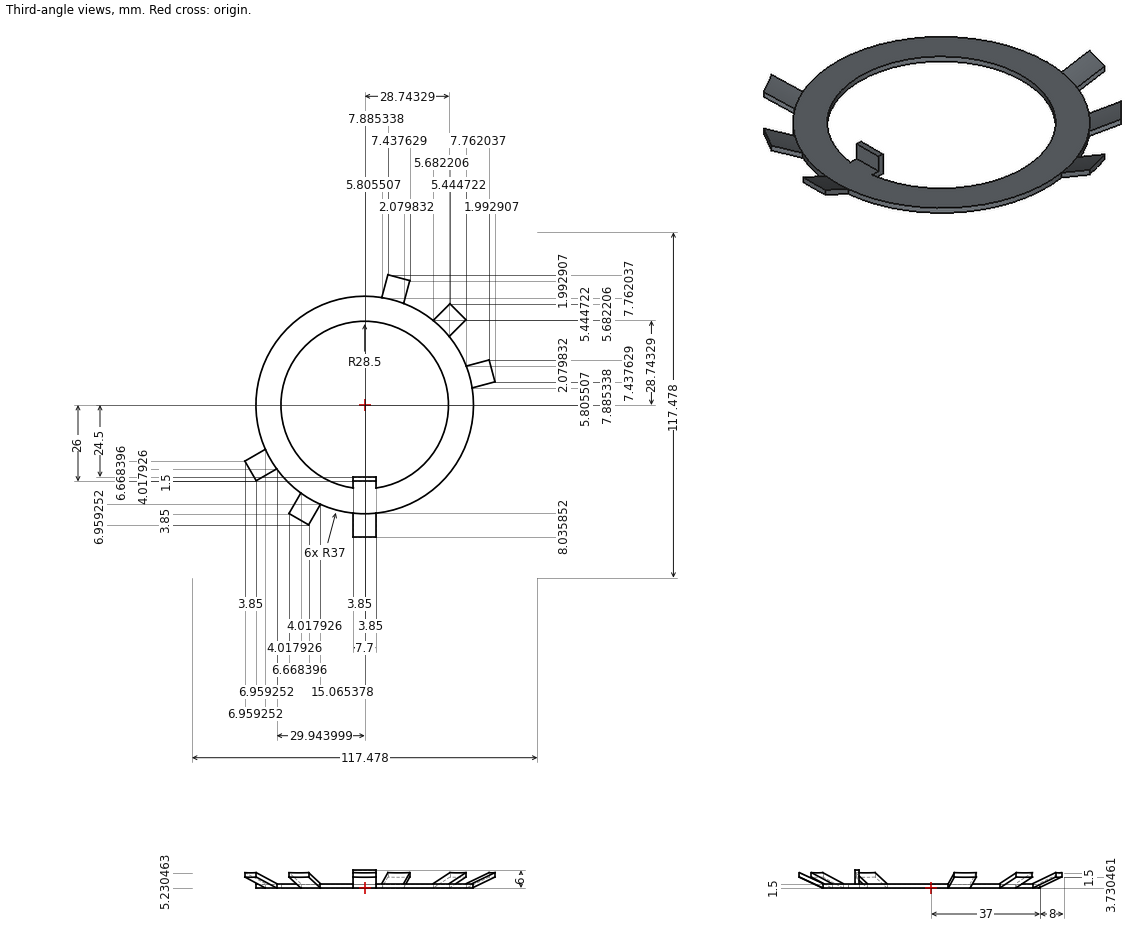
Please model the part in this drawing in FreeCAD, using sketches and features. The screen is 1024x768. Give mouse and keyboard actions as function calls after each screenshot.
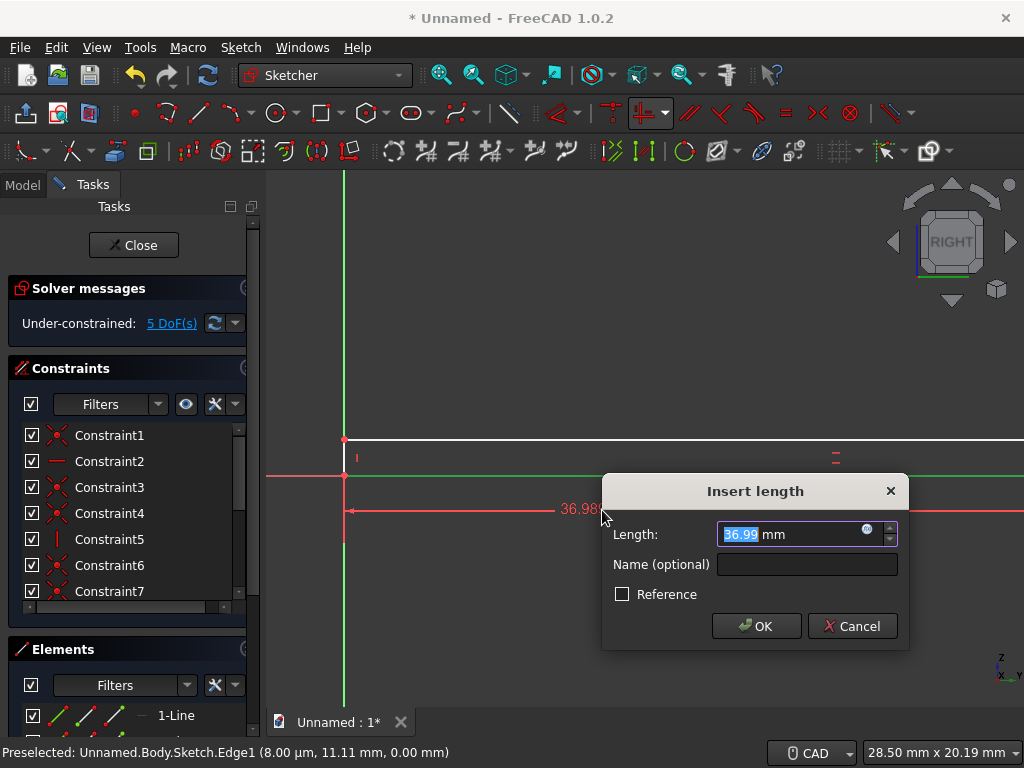
text(37)
key(Return)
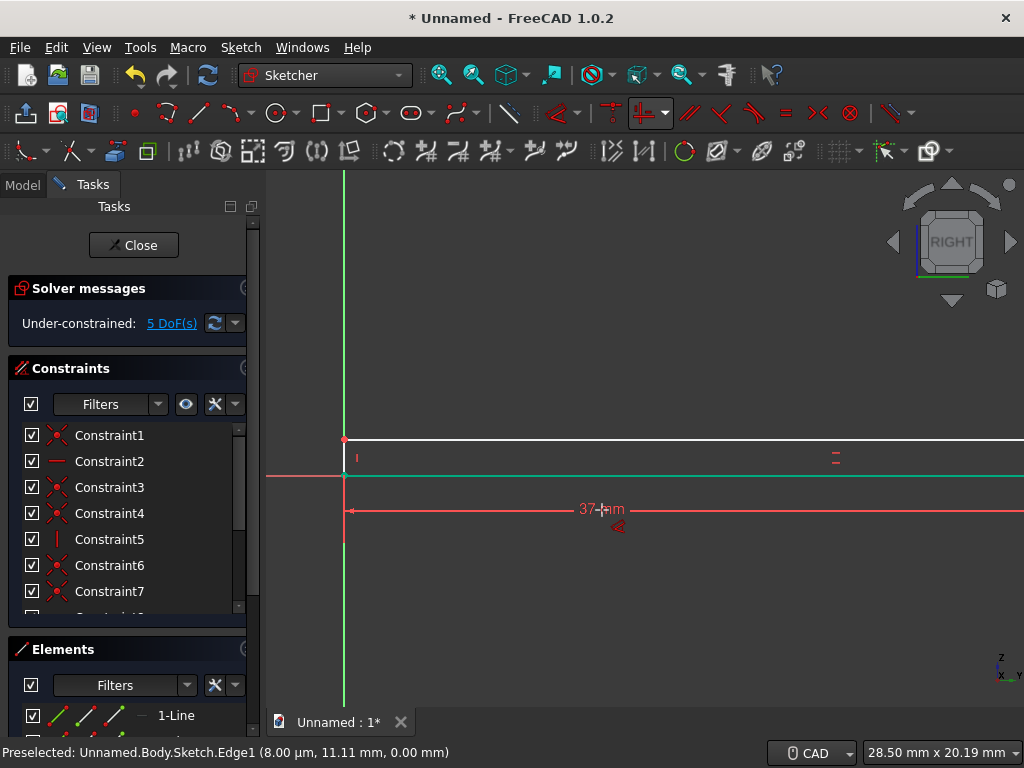
click(640, 439)
click(602, 405)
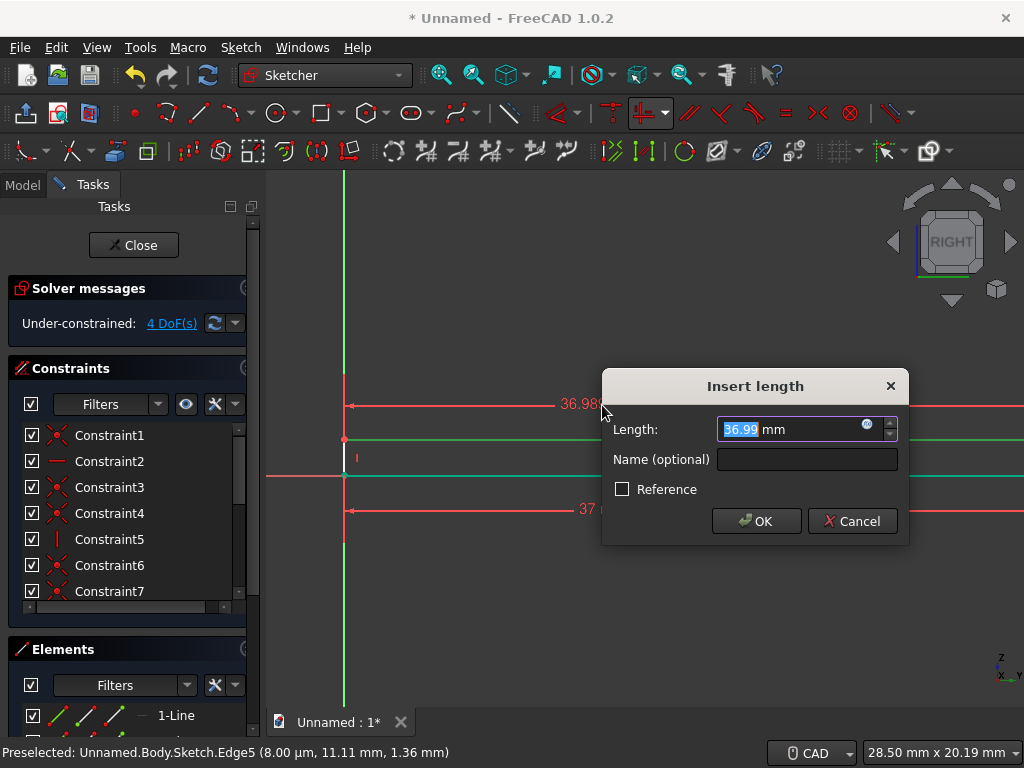
text(37)
key(Return)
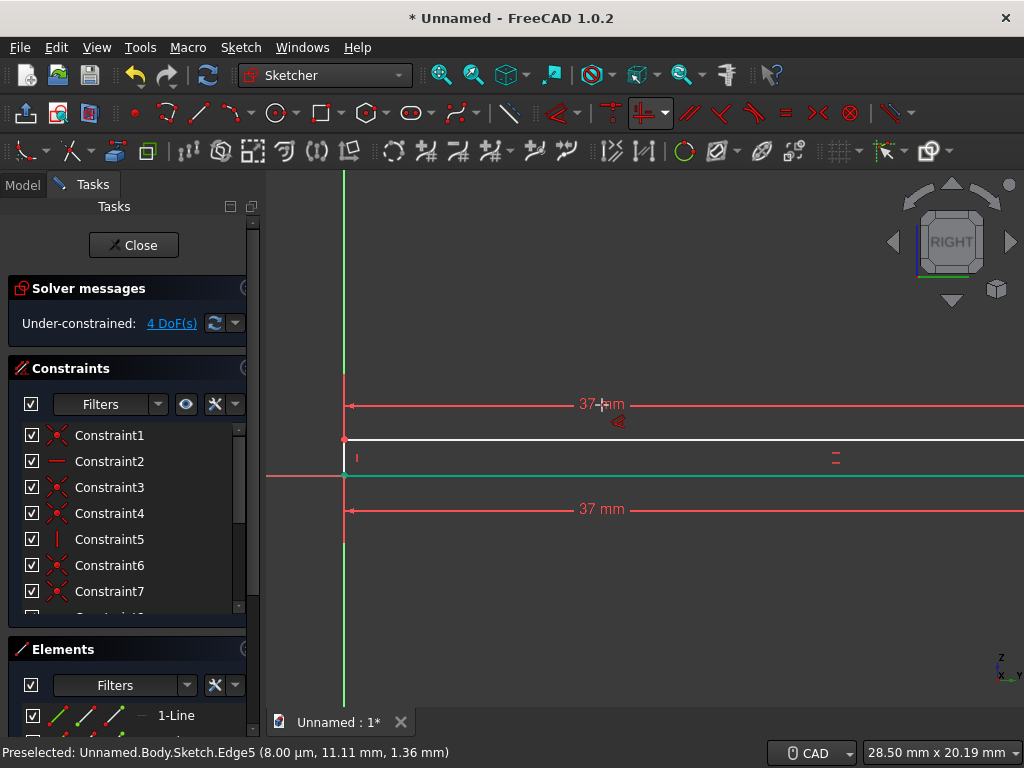
scroll(363, 457, down, 5)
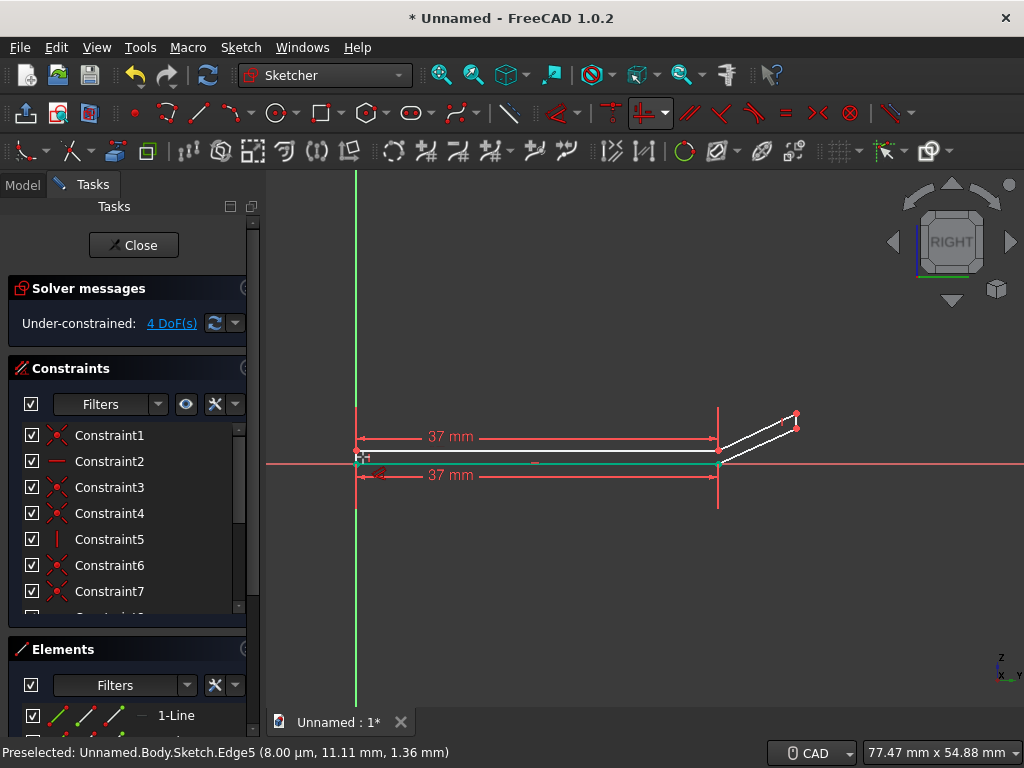
scroll(742, 454, up, 2)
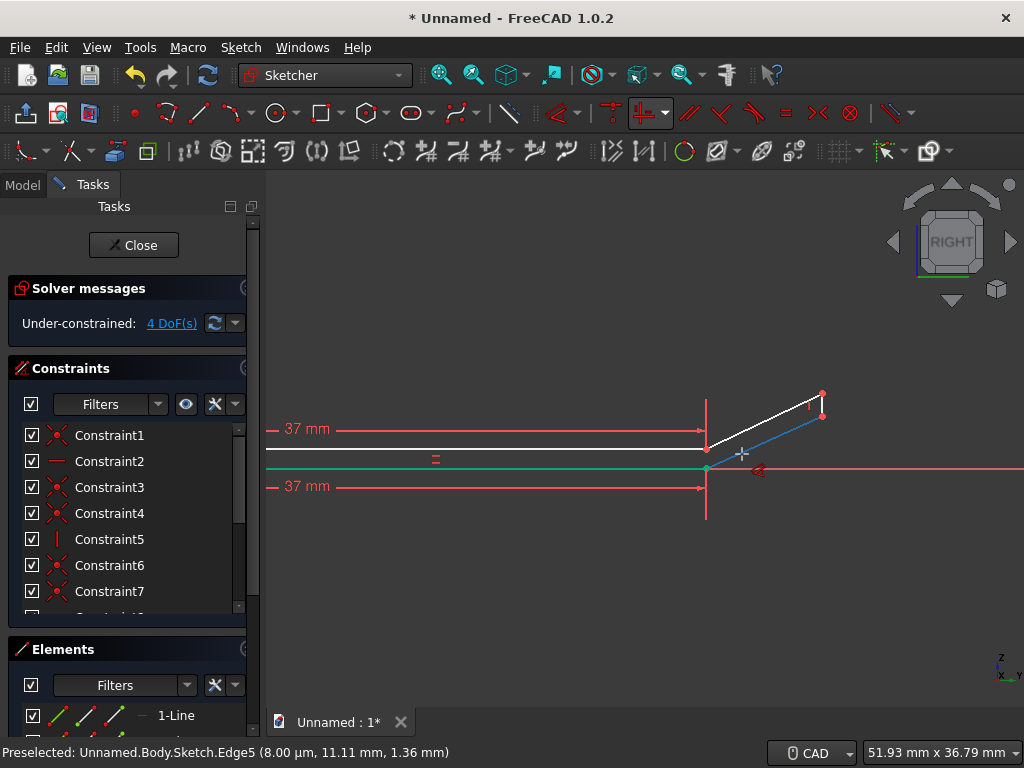
click(741, 453)
click(764, 503)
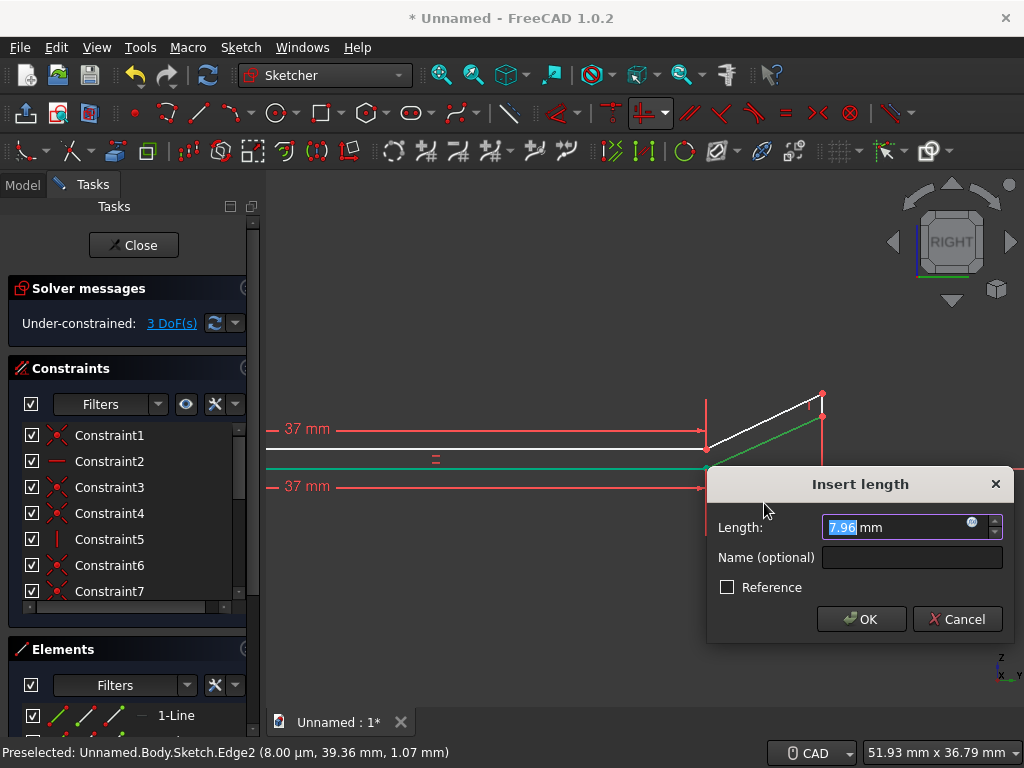
text(8)
key(Return)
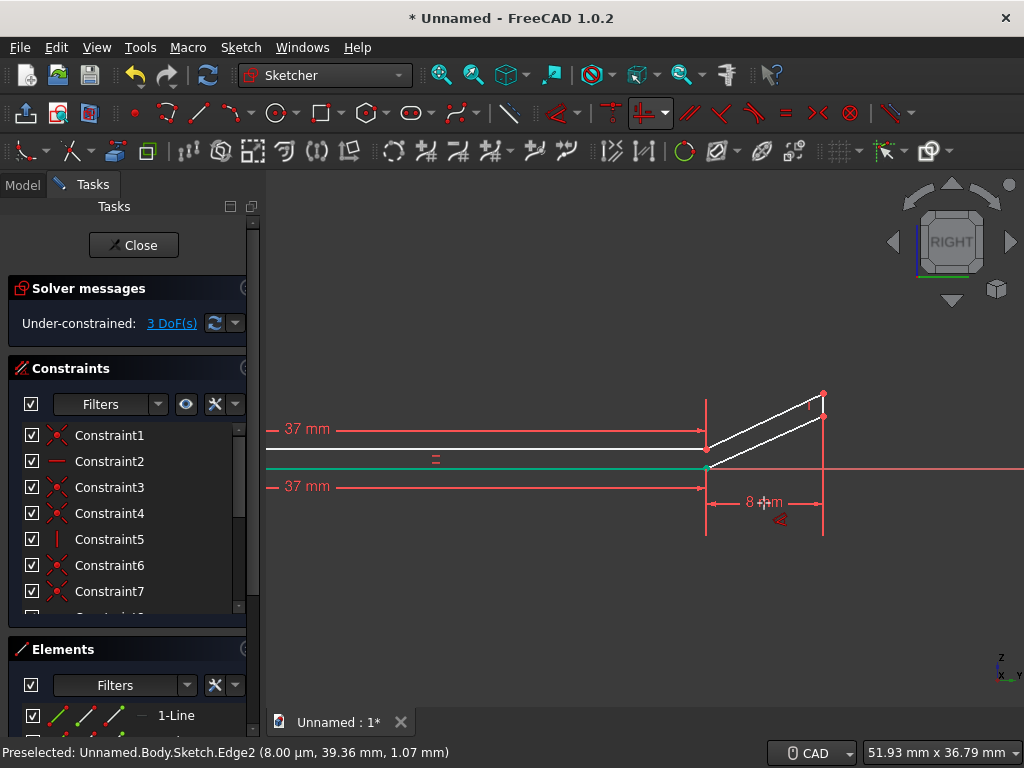
scroll(823, 405, up, 3)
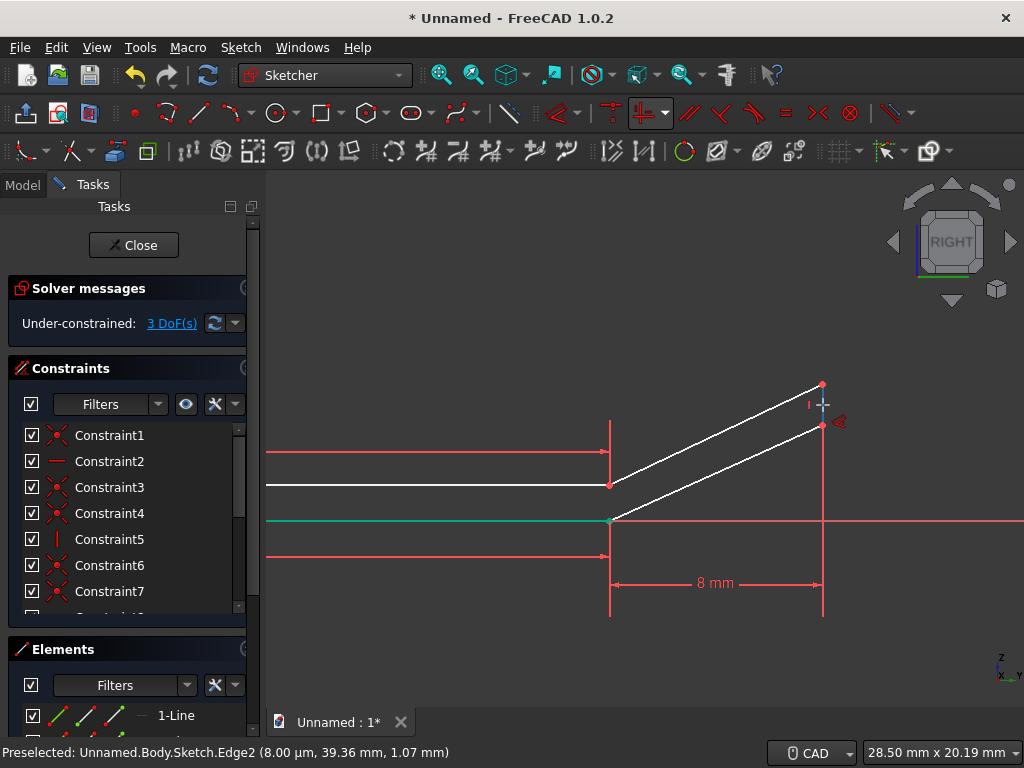
click(823, 405)
click(857, 405)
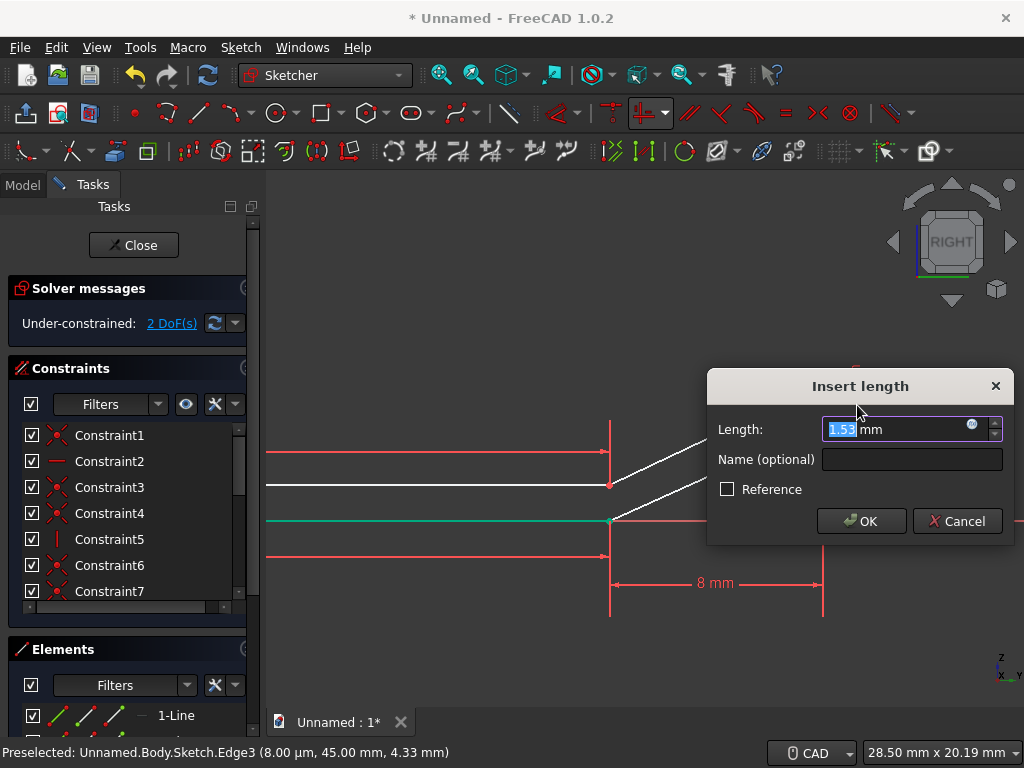
text(1.5)
key(Return)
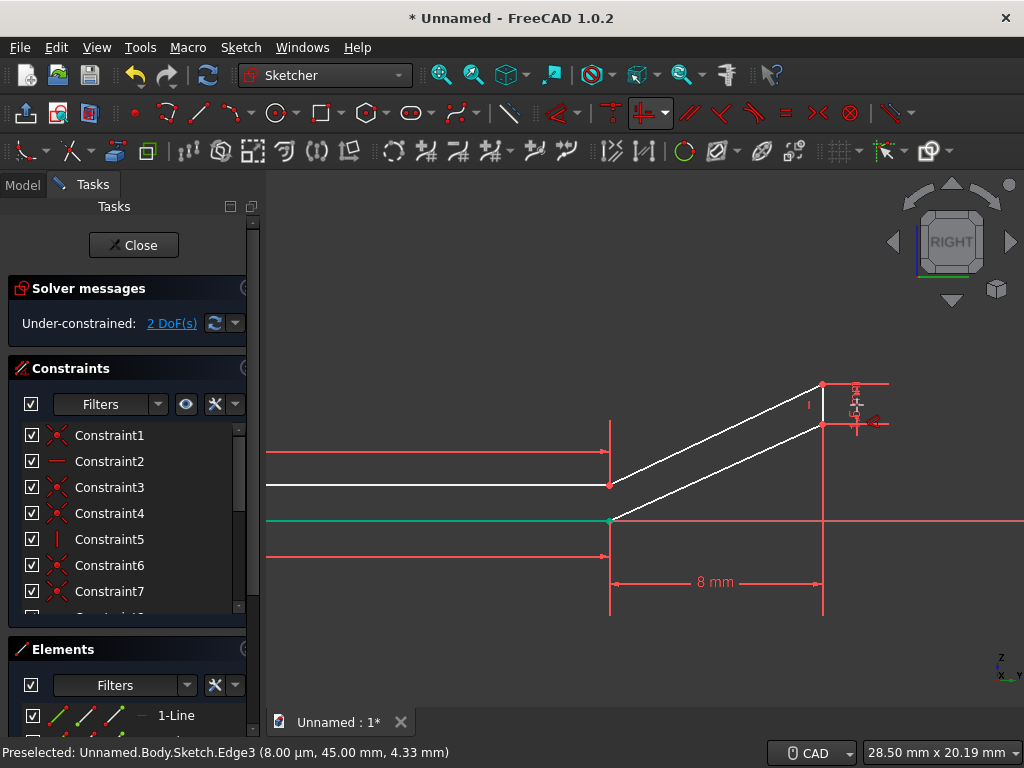
scroll(782, 431, down, 5)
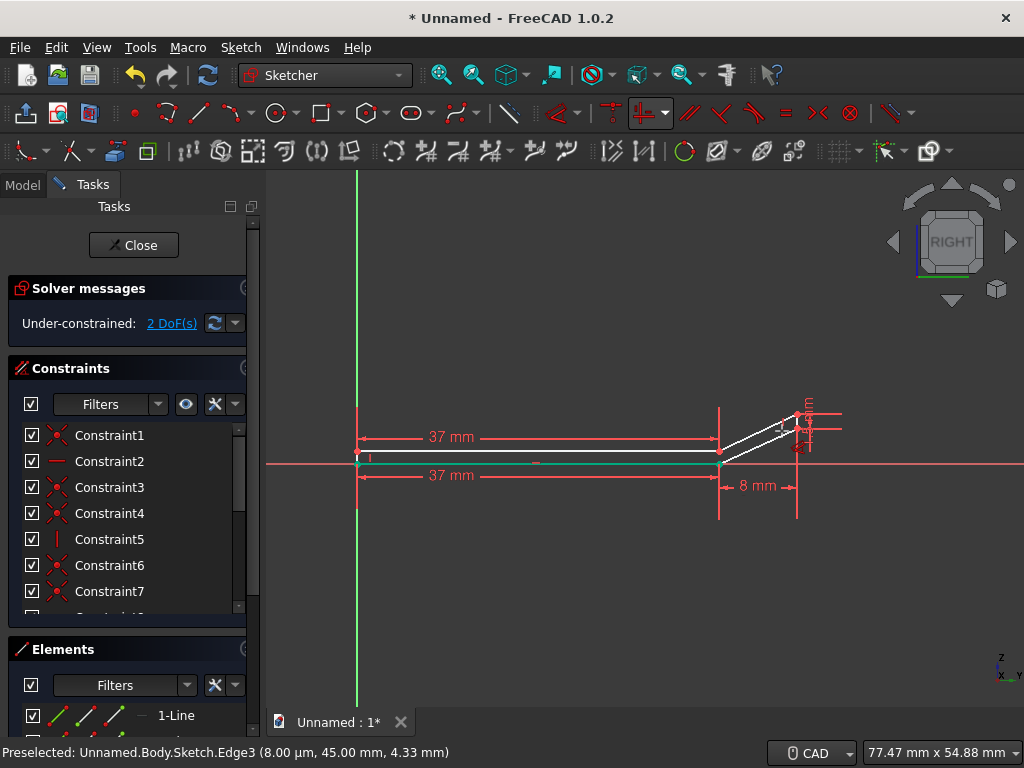
scroll(357, 455, up, 7)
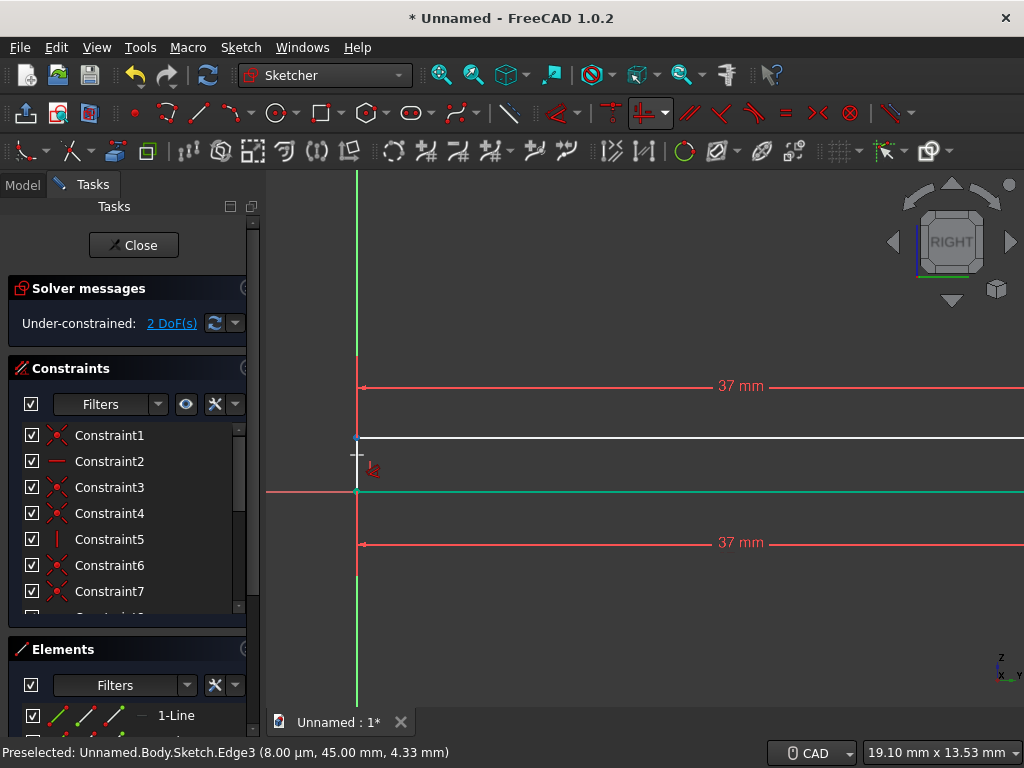
click(357, 454)
click(323, 465)